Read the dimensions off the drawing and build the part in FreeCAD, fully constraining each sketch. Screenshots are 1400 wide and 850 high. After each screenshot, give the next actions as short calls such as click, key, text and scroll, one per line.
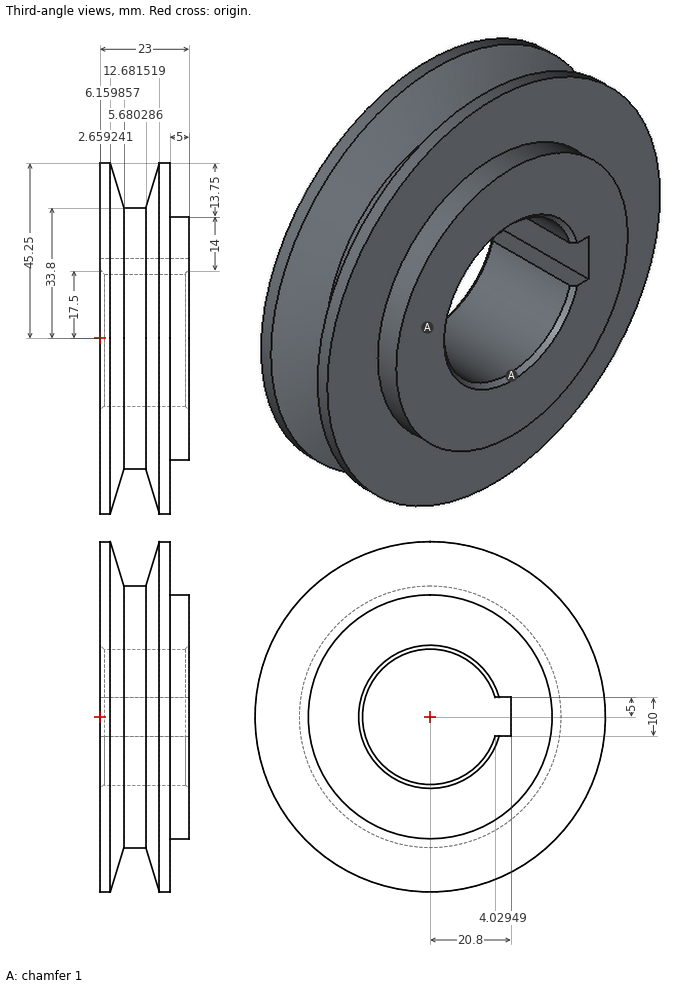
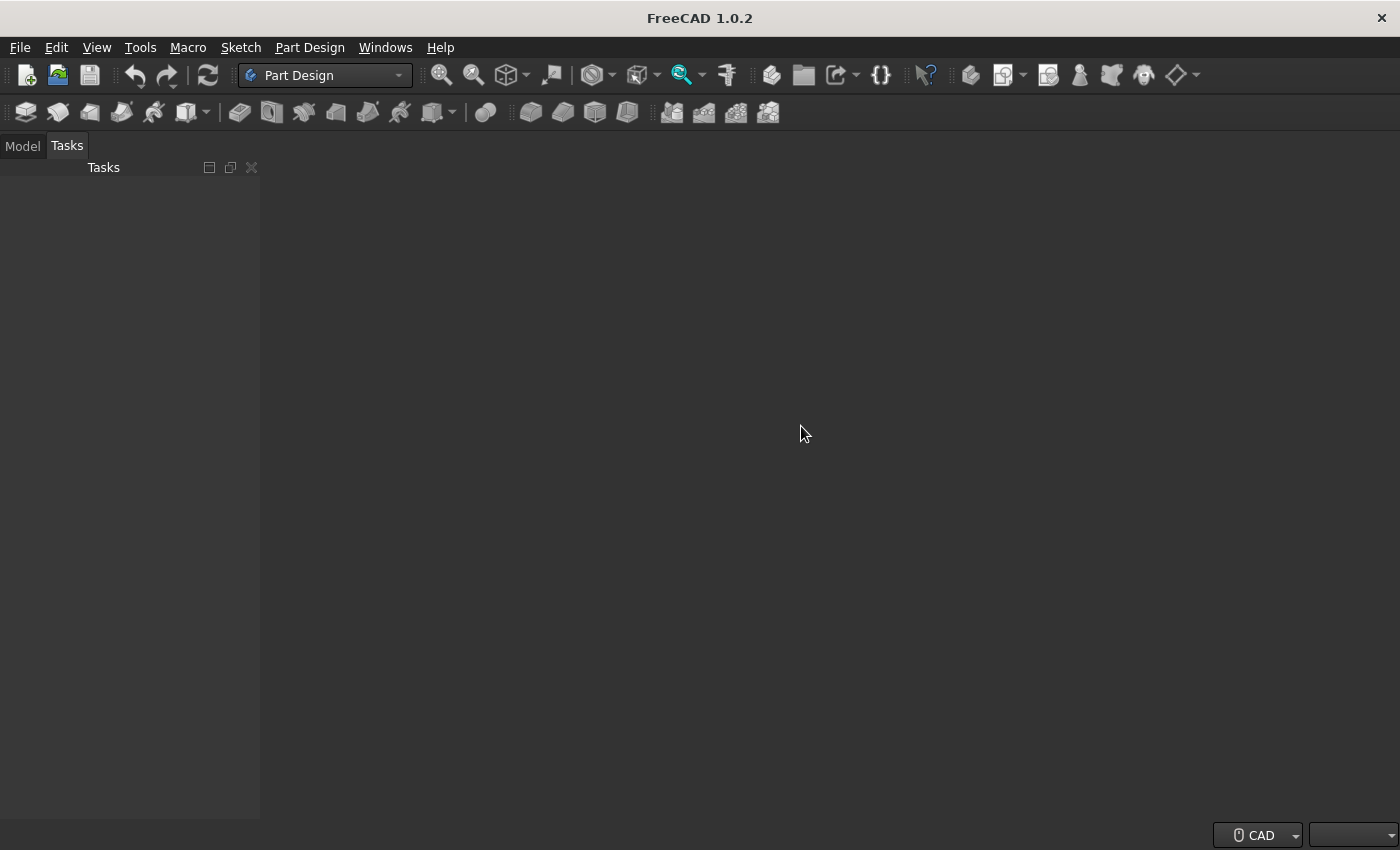
key(ctrl+n)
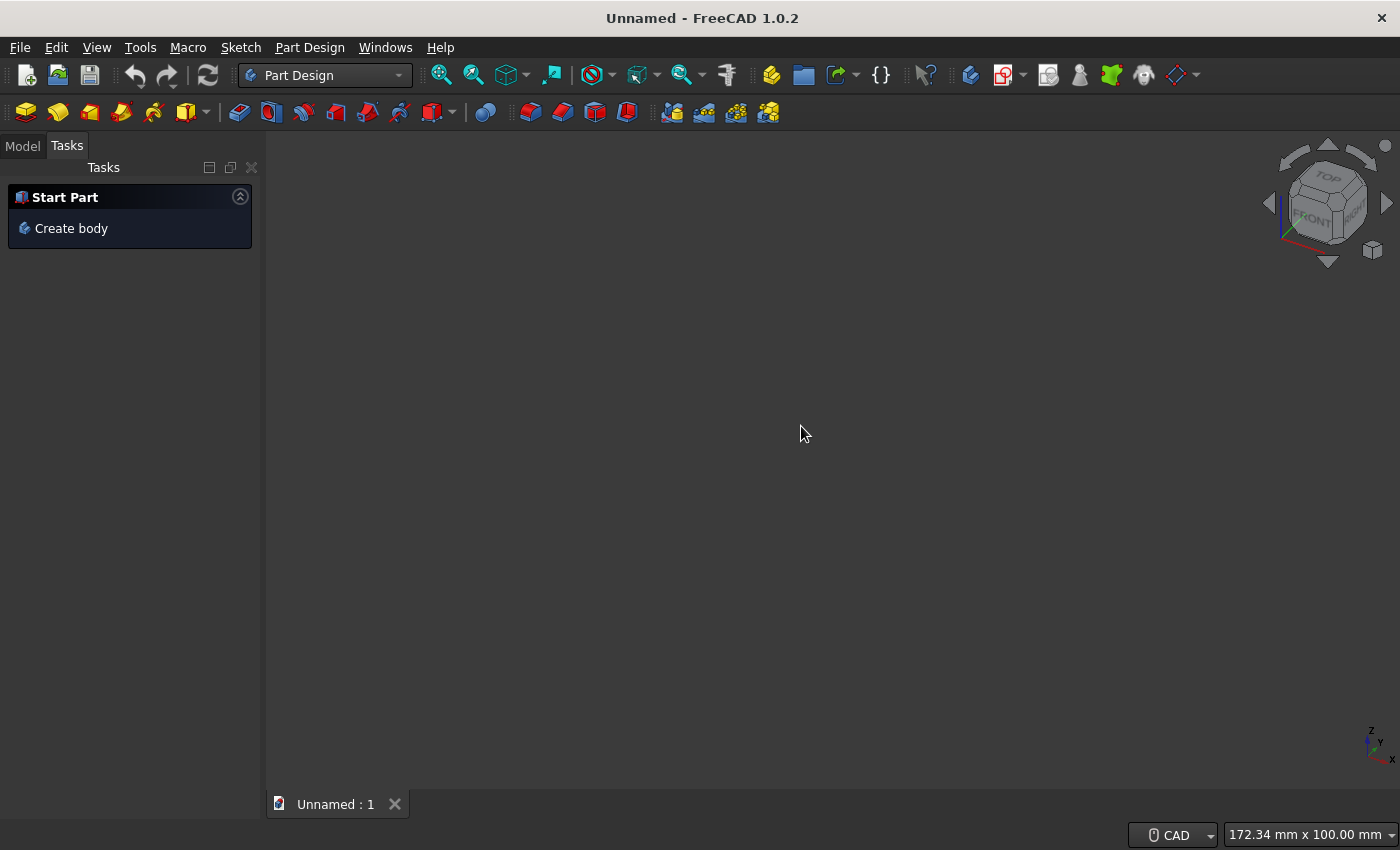
click(1004, 76)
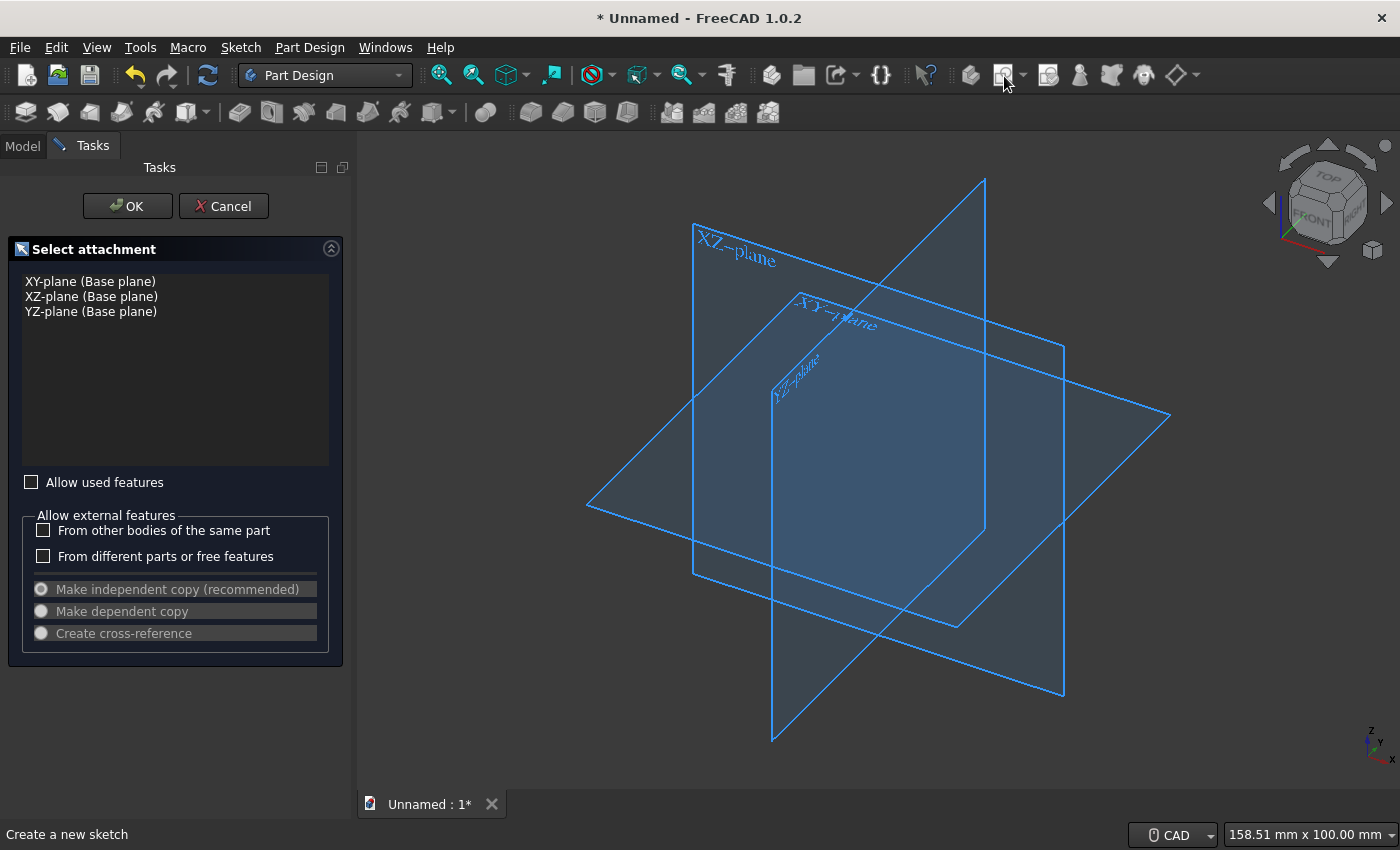
click(82, 282)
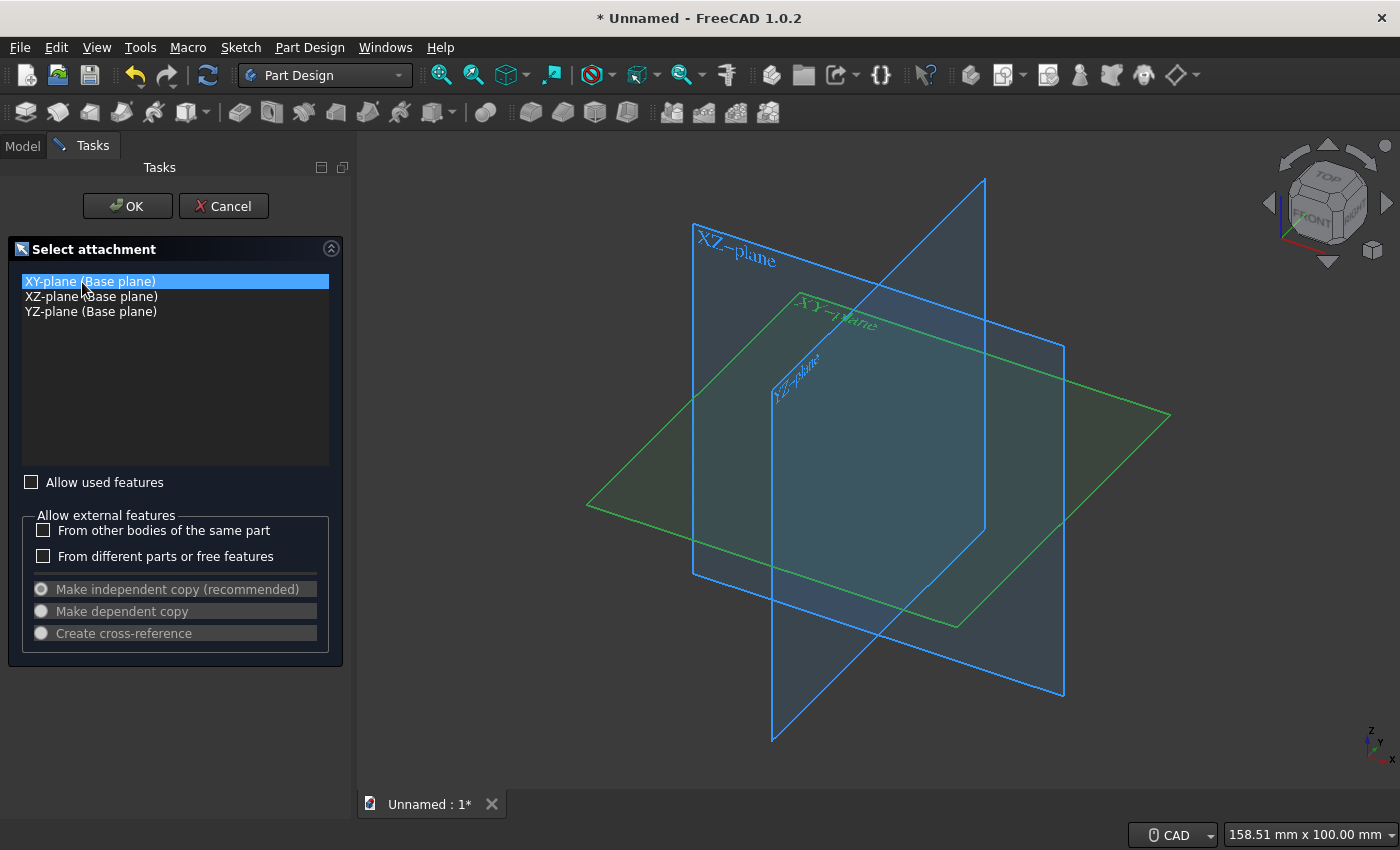
click(128, 206)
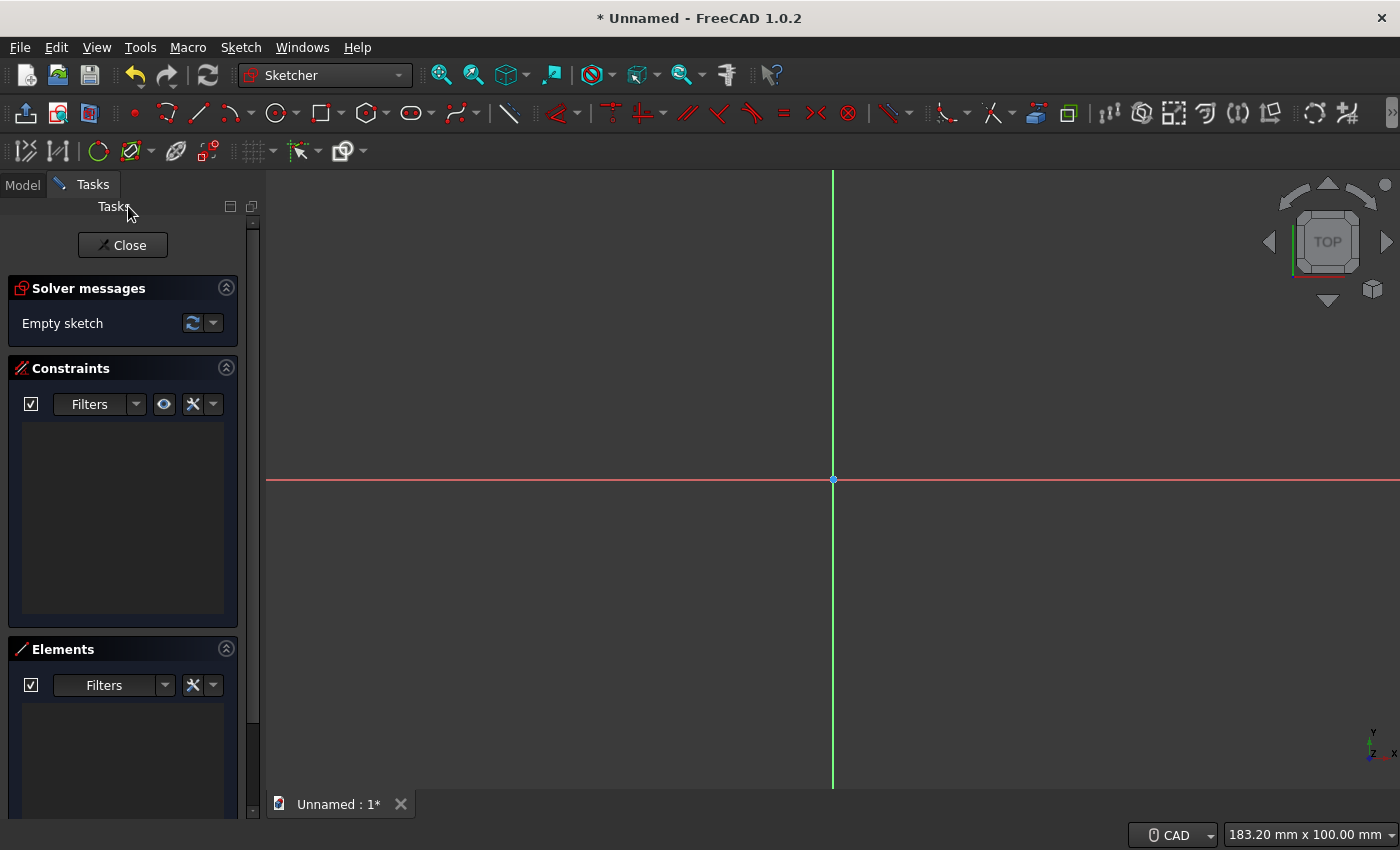
scroll(294, 761, down, 1)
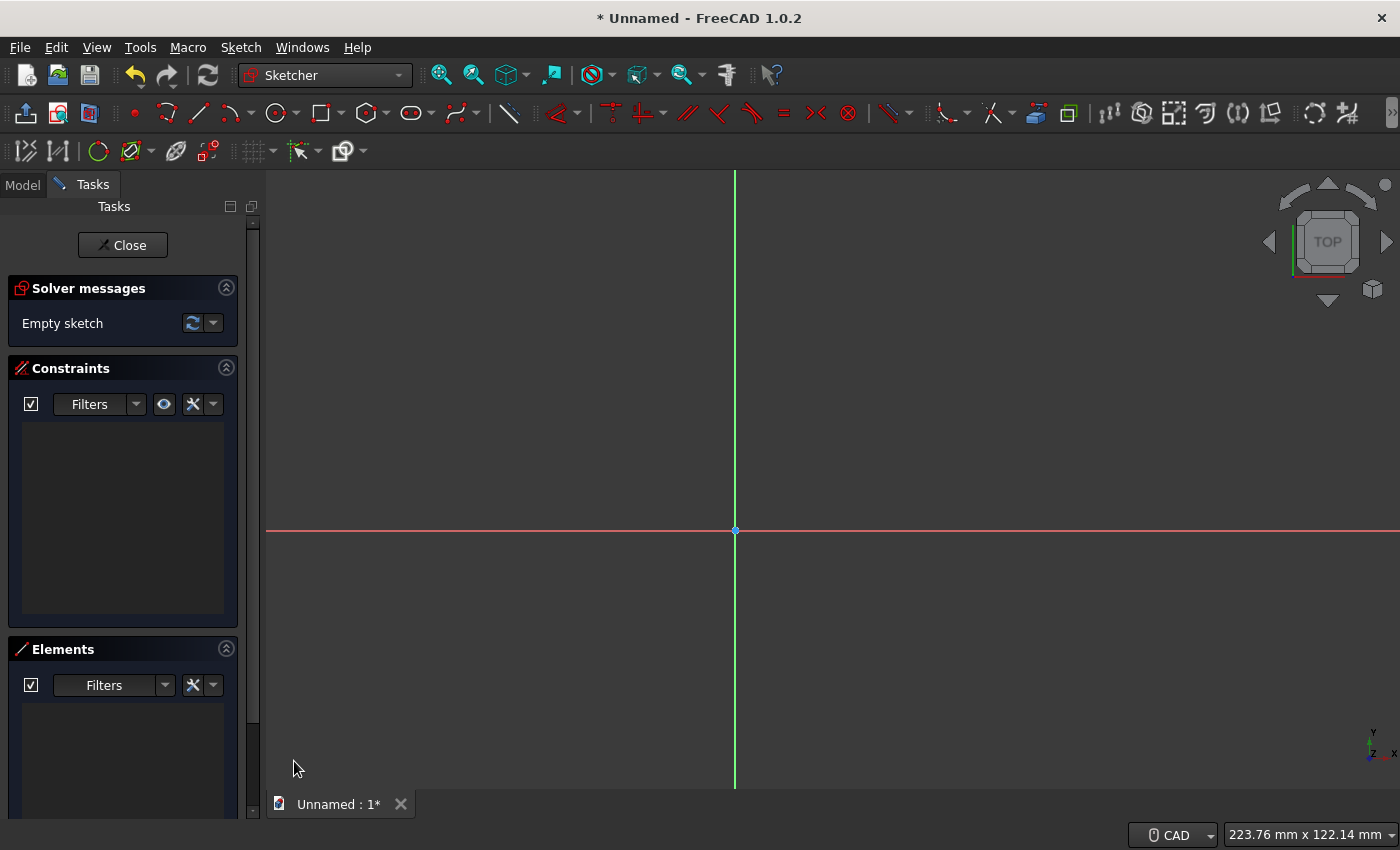
scroll(829, 339, up, 3)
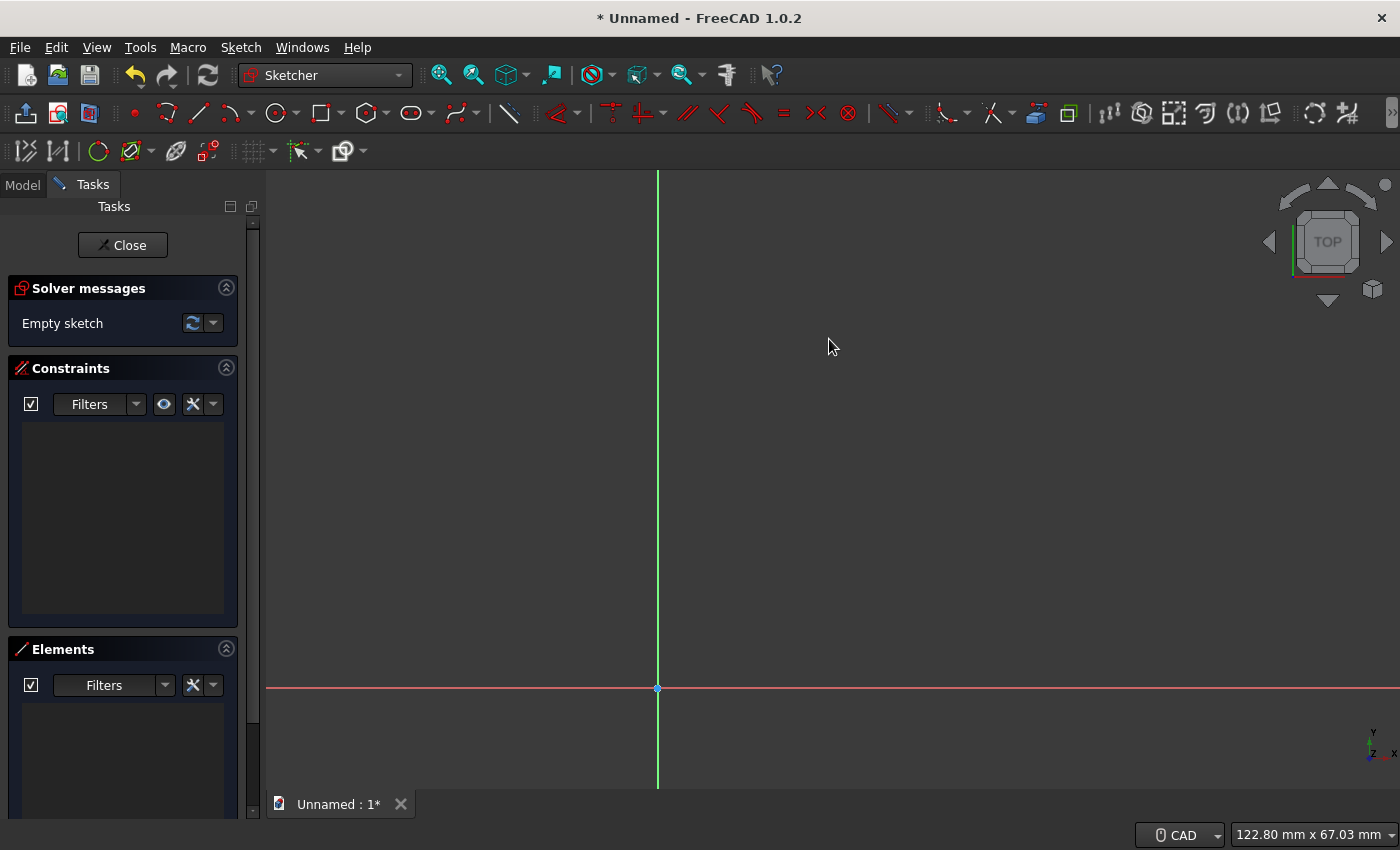
key(g)
key(m)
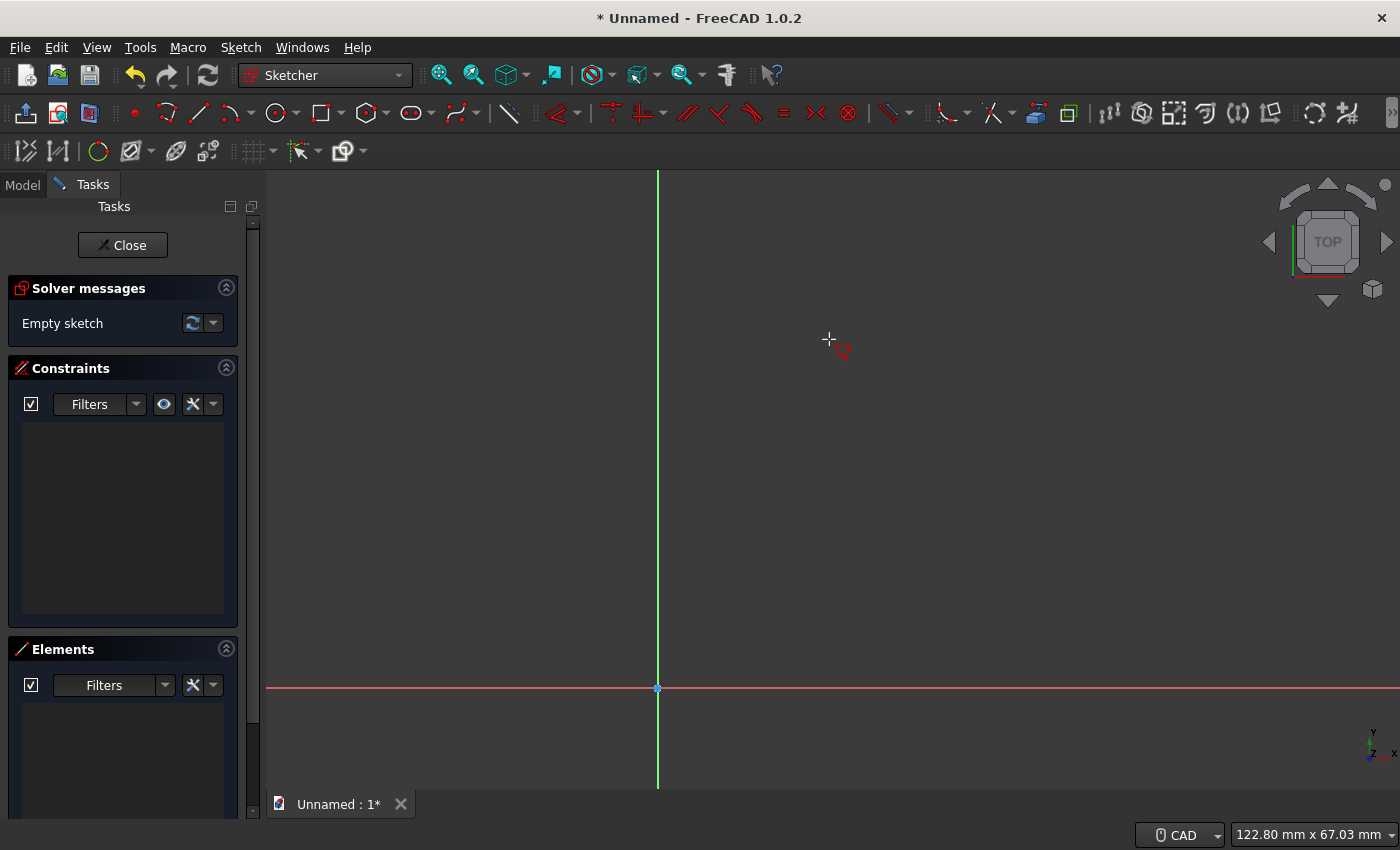
click(658, 526)
click(870, 526)
click(870, 397)
click(824, 397)
click(824, 270)
click(667, 270)
click(658, 527)
key(Escape)
key(Escape)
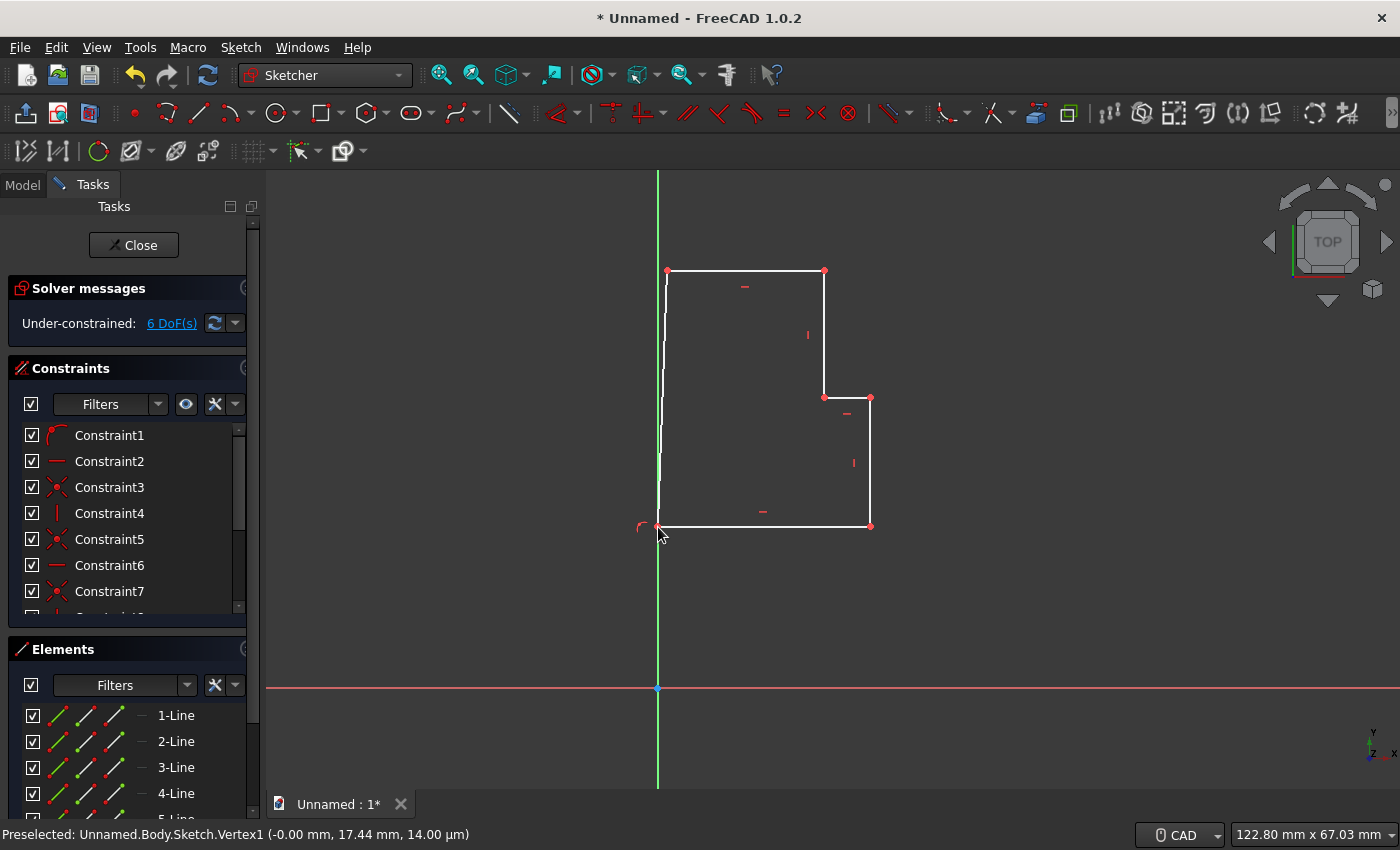
click(661, 450)